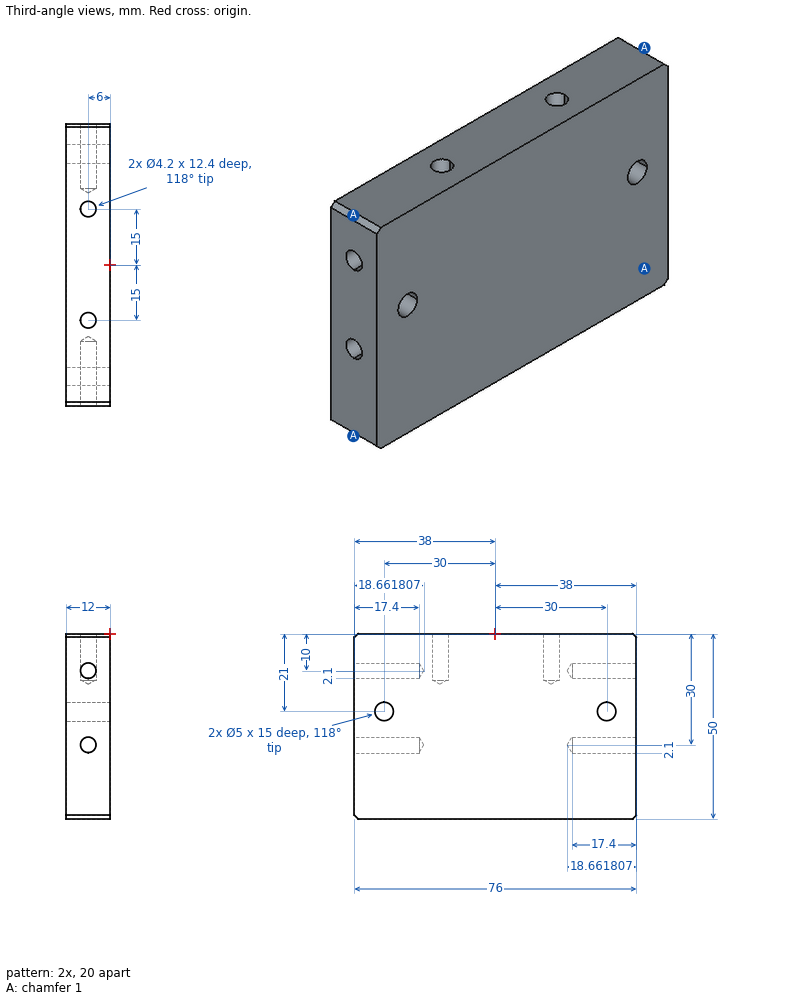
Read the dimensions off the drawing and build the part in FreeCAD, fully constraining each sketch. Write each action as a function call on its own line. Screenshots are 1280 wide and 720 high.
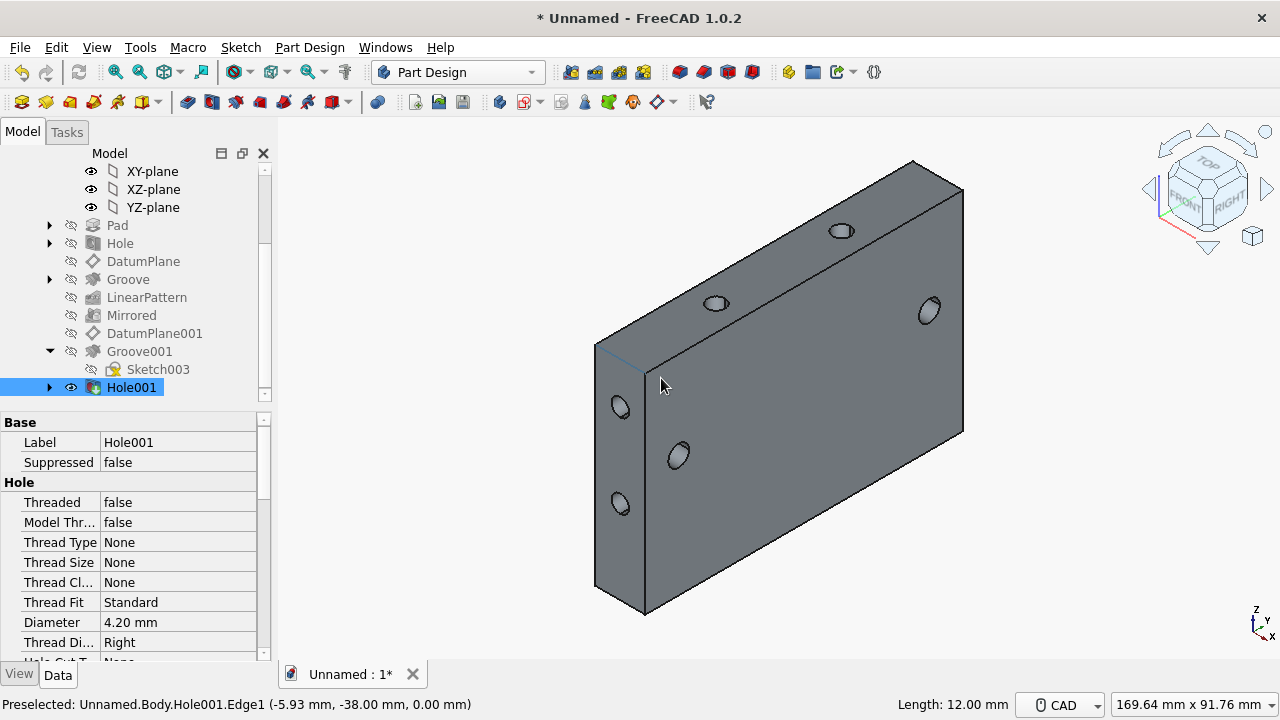
key(2)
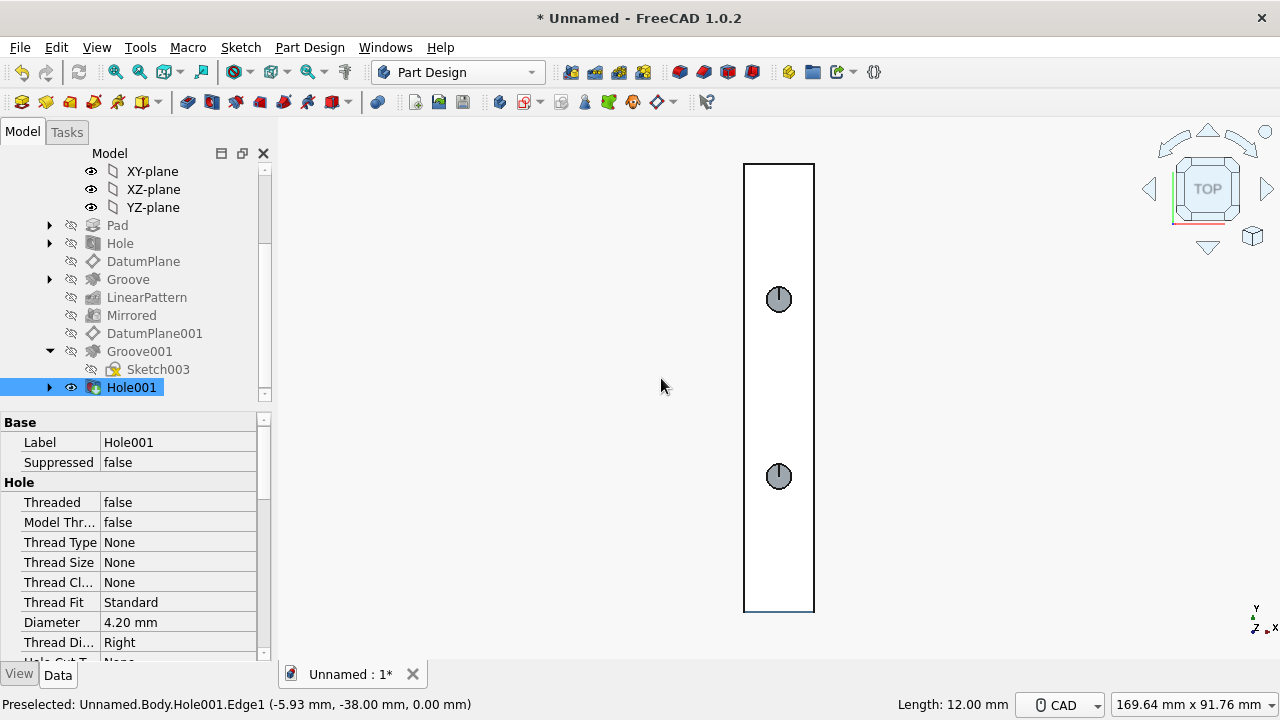
key(1)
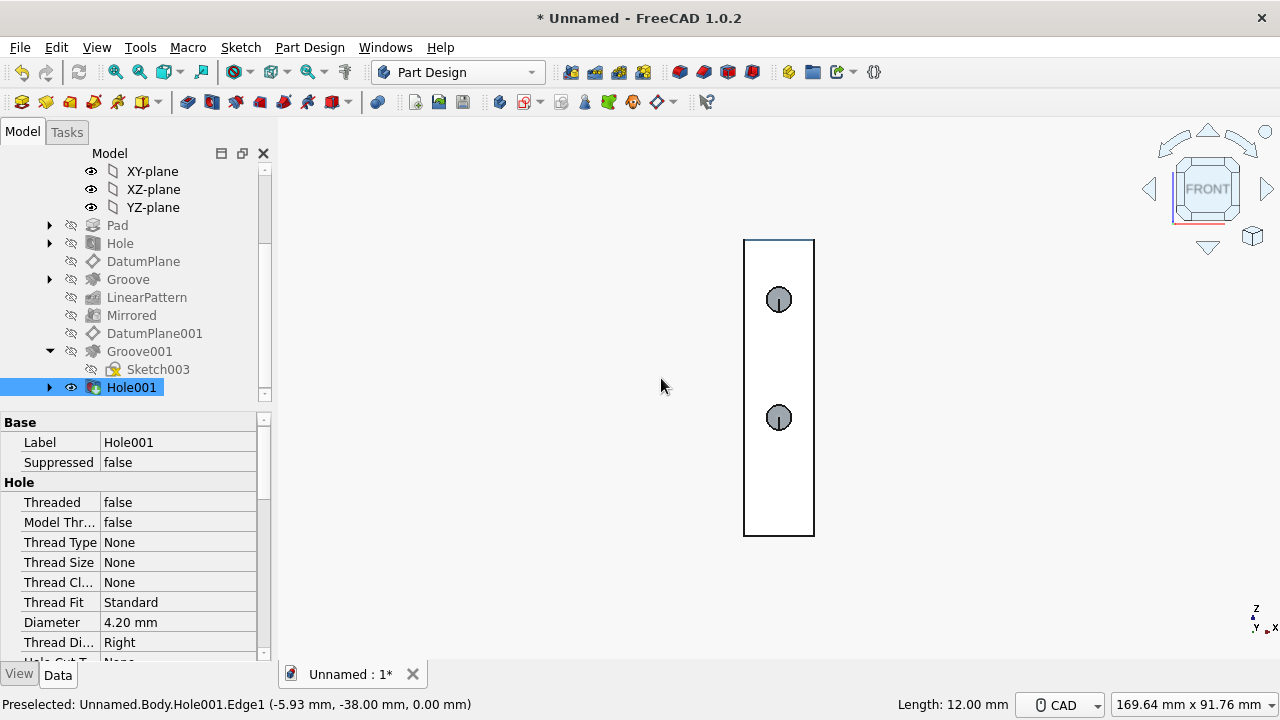
click(779, 535, ctrl)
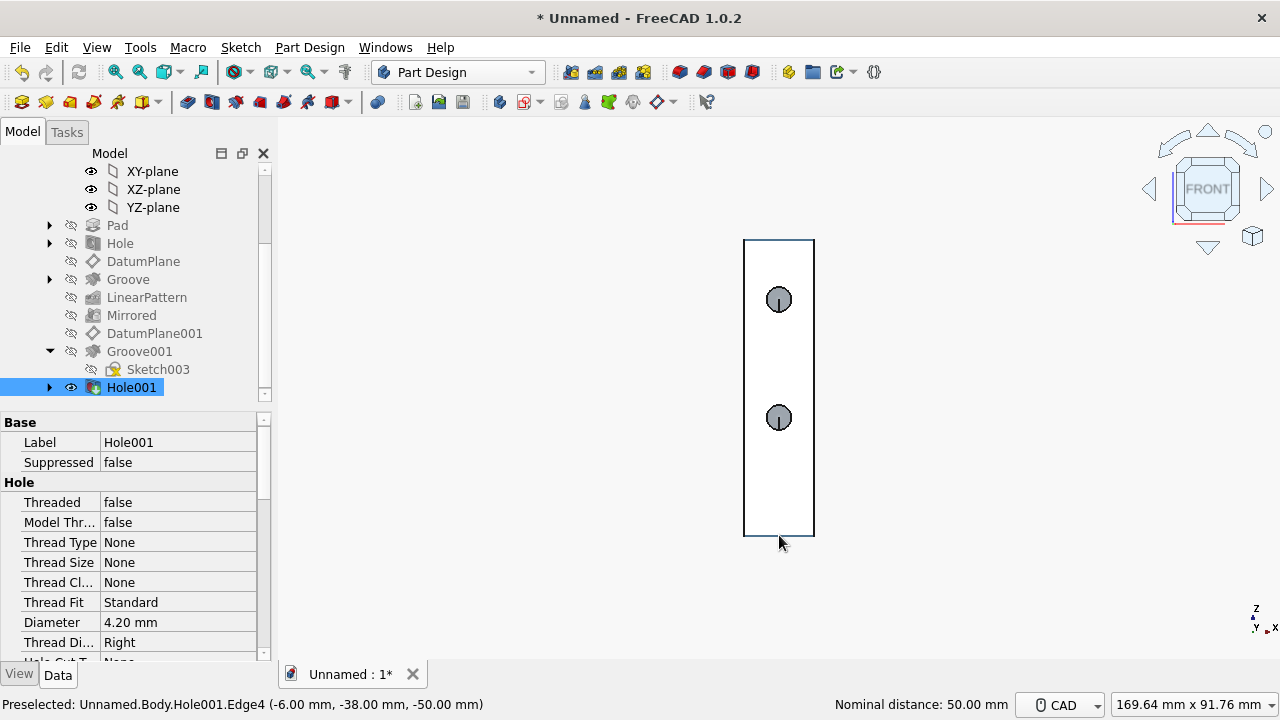
key(3)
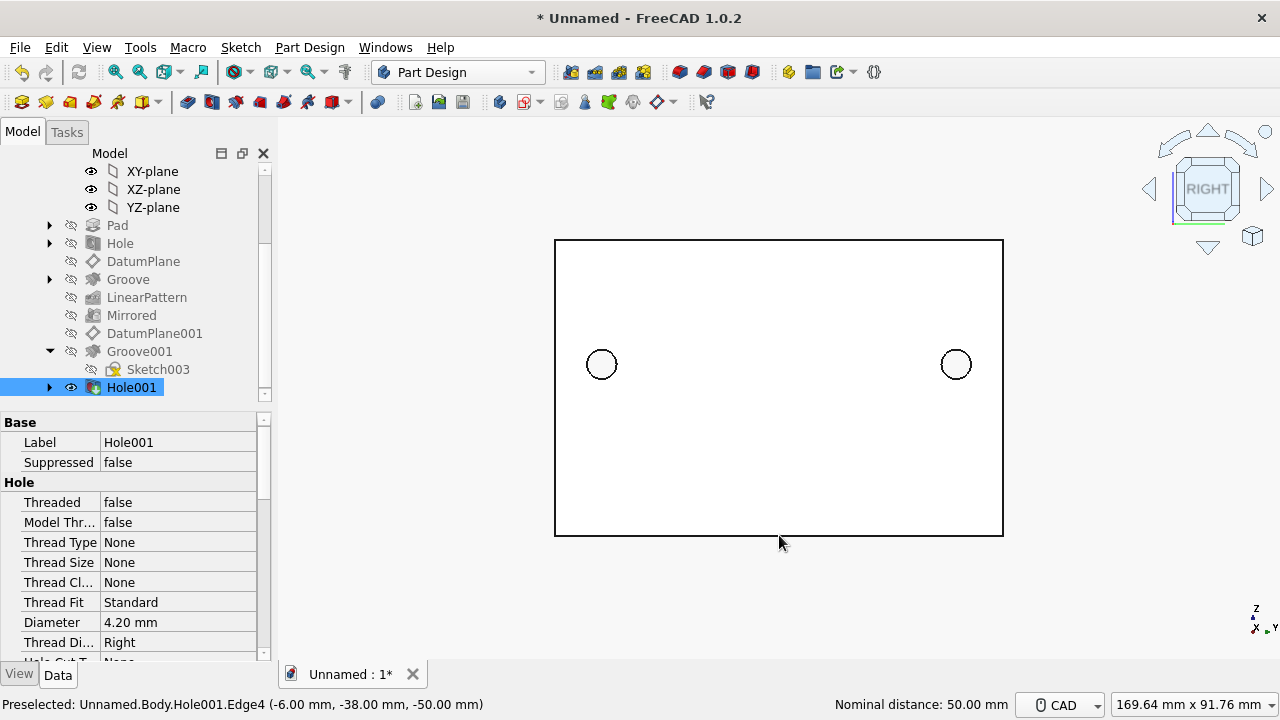
key(5)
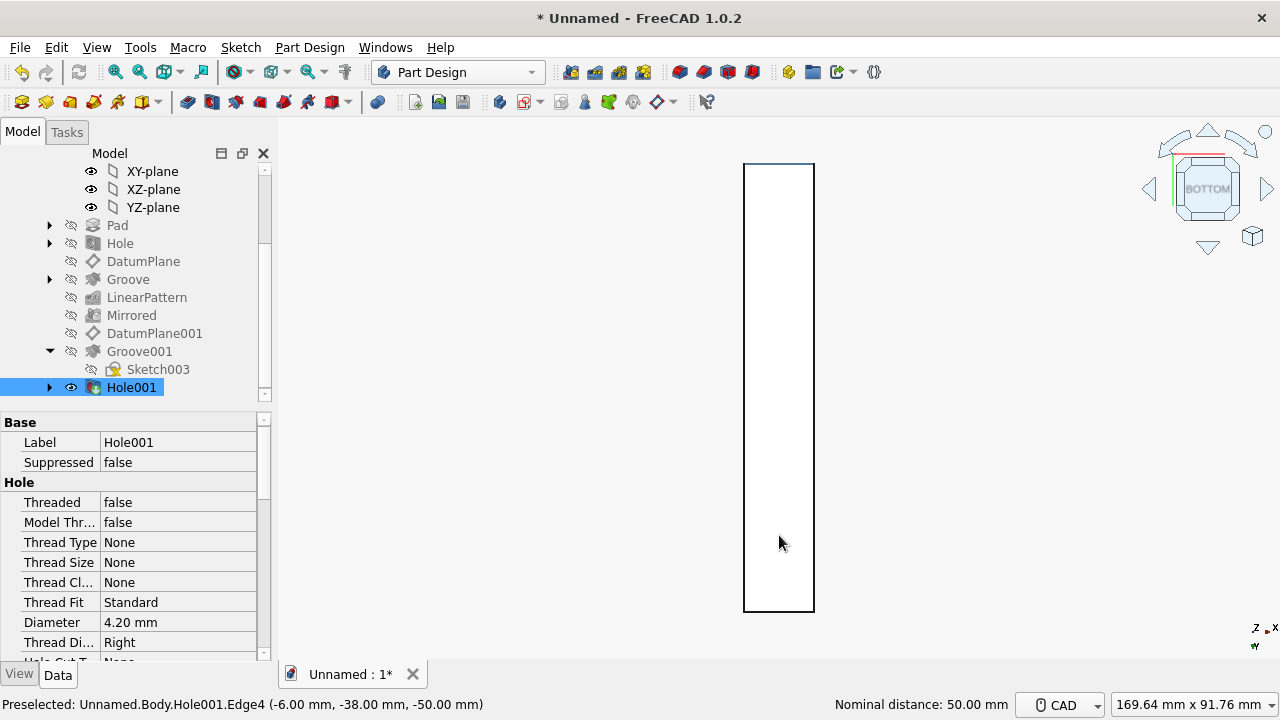
click(779, 611, ctrl)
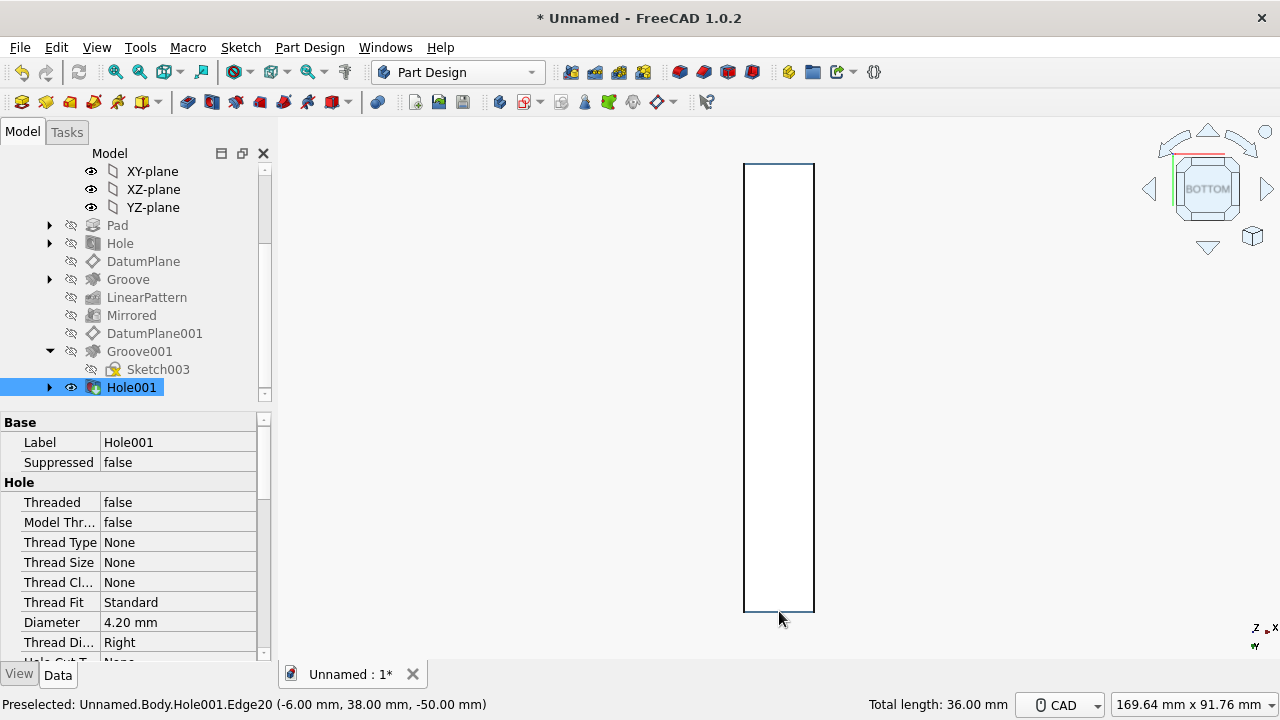
key(4)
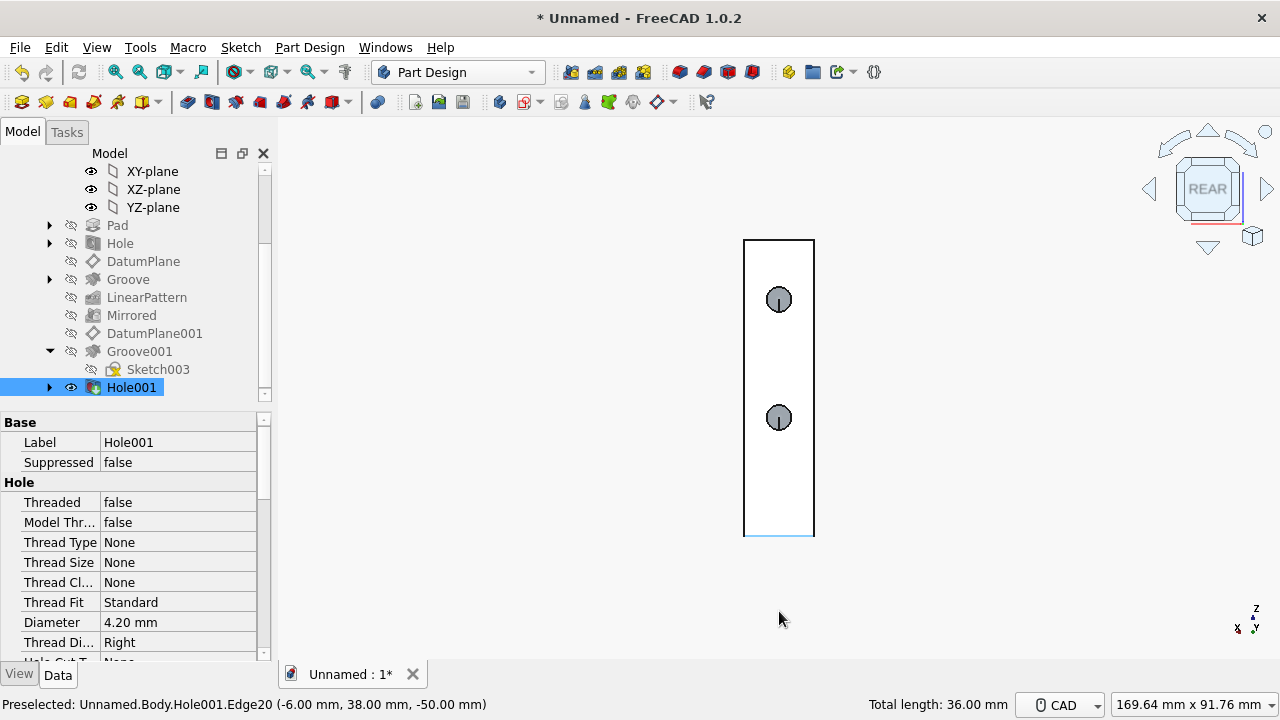
click(779, 239, ctrl)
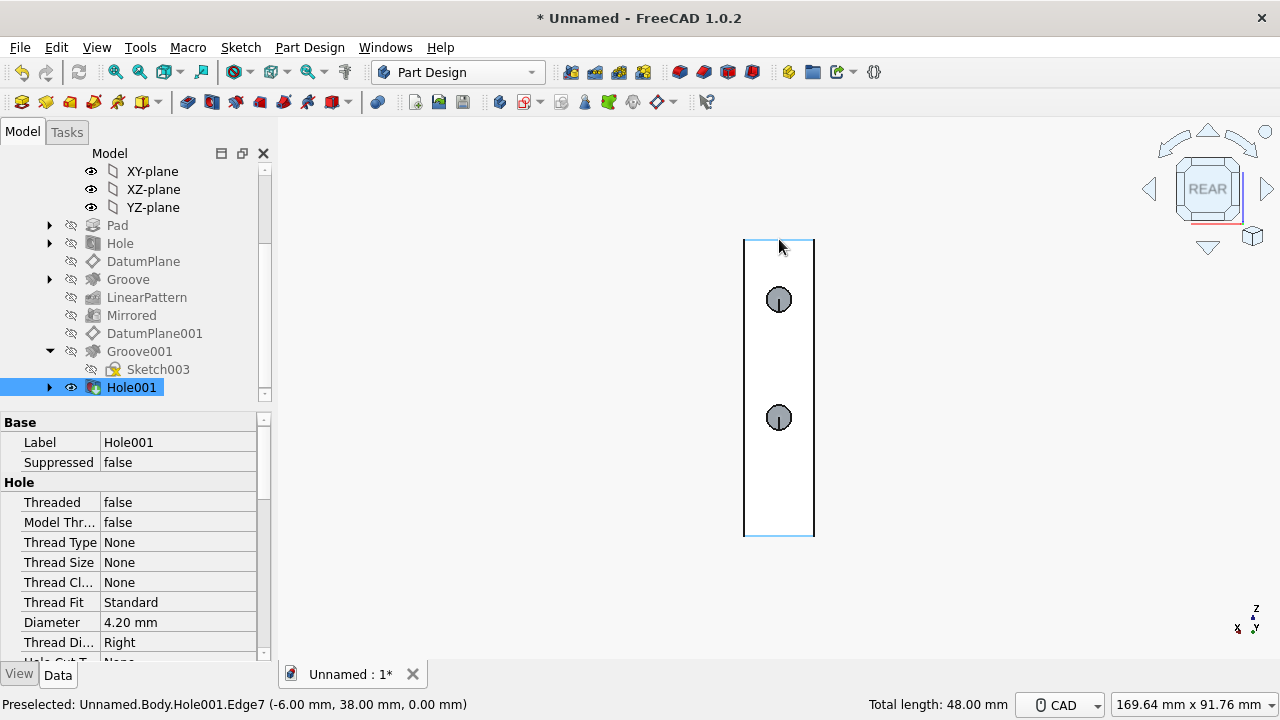
click(704, 72)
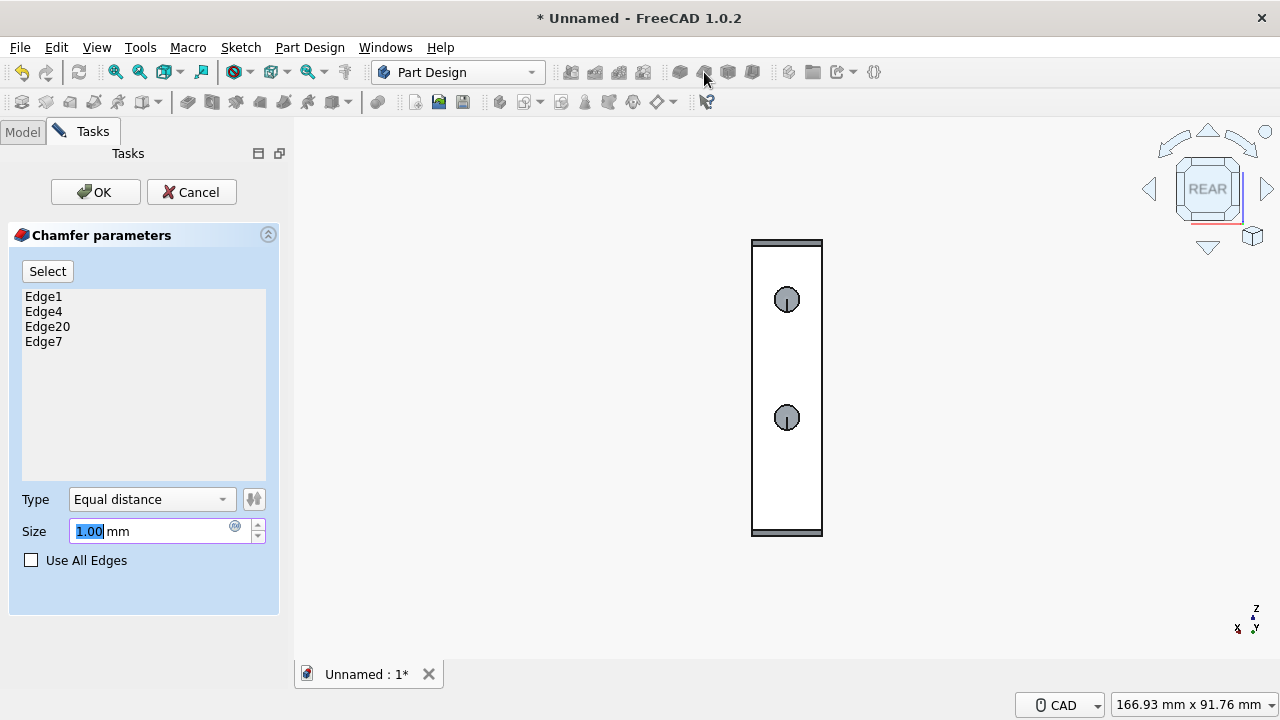
text(1)
key(Tab)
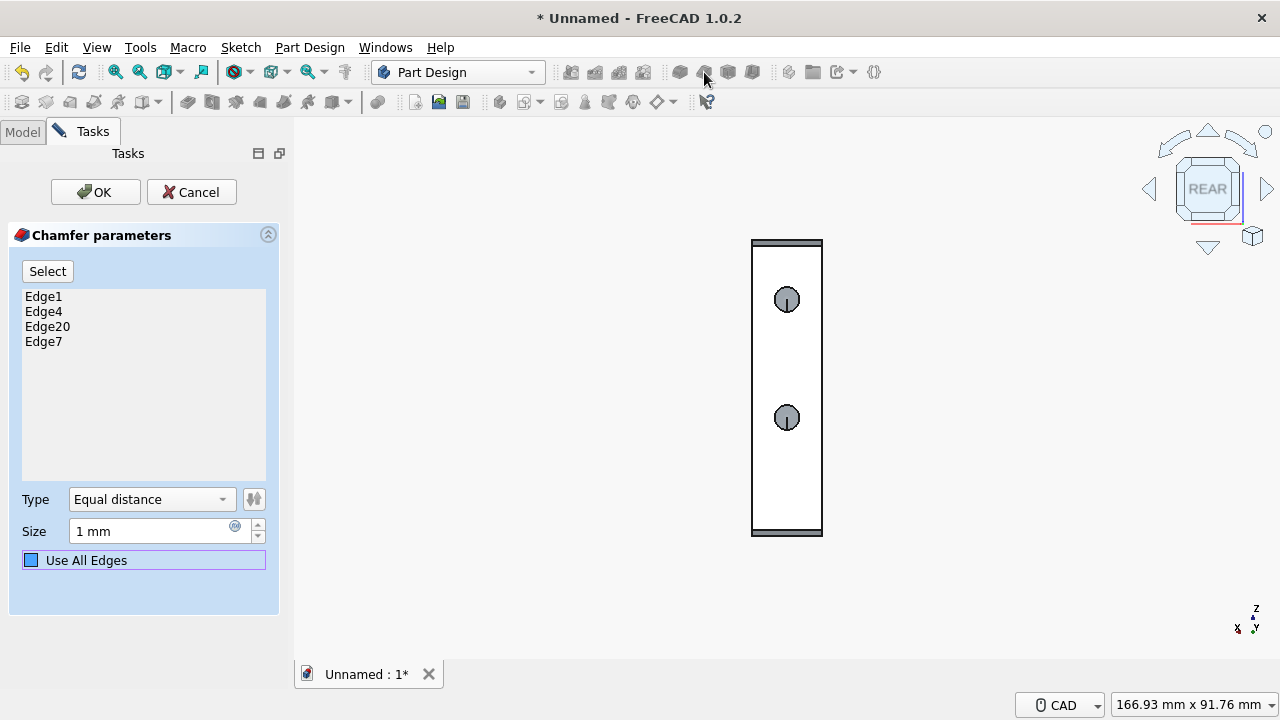
click(96, 192)